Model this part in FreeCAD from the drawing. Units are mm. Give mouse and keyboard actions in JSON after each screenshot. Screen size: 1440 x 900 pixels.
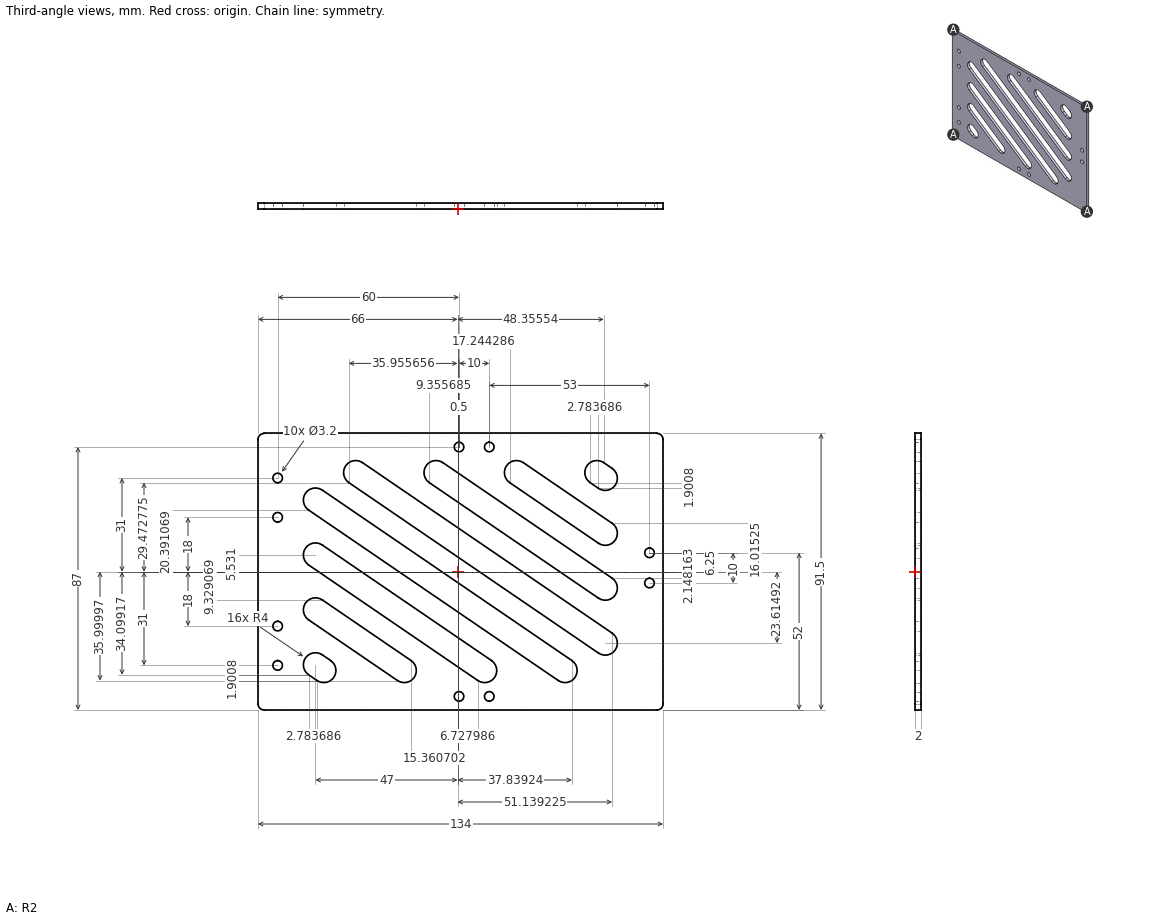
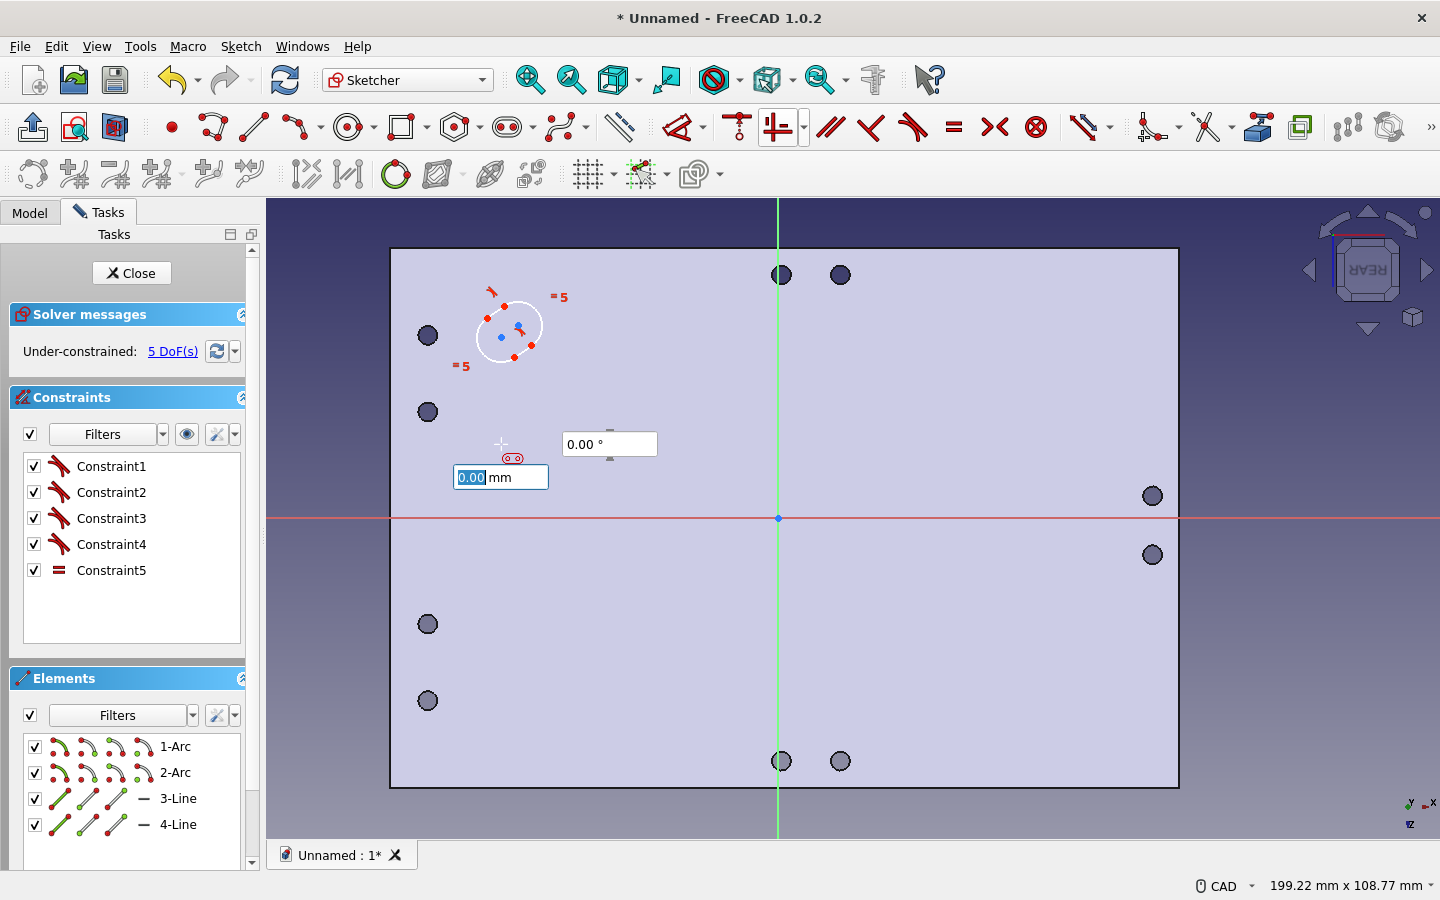
{"action": "left_click", "coordinate": [675, 325]}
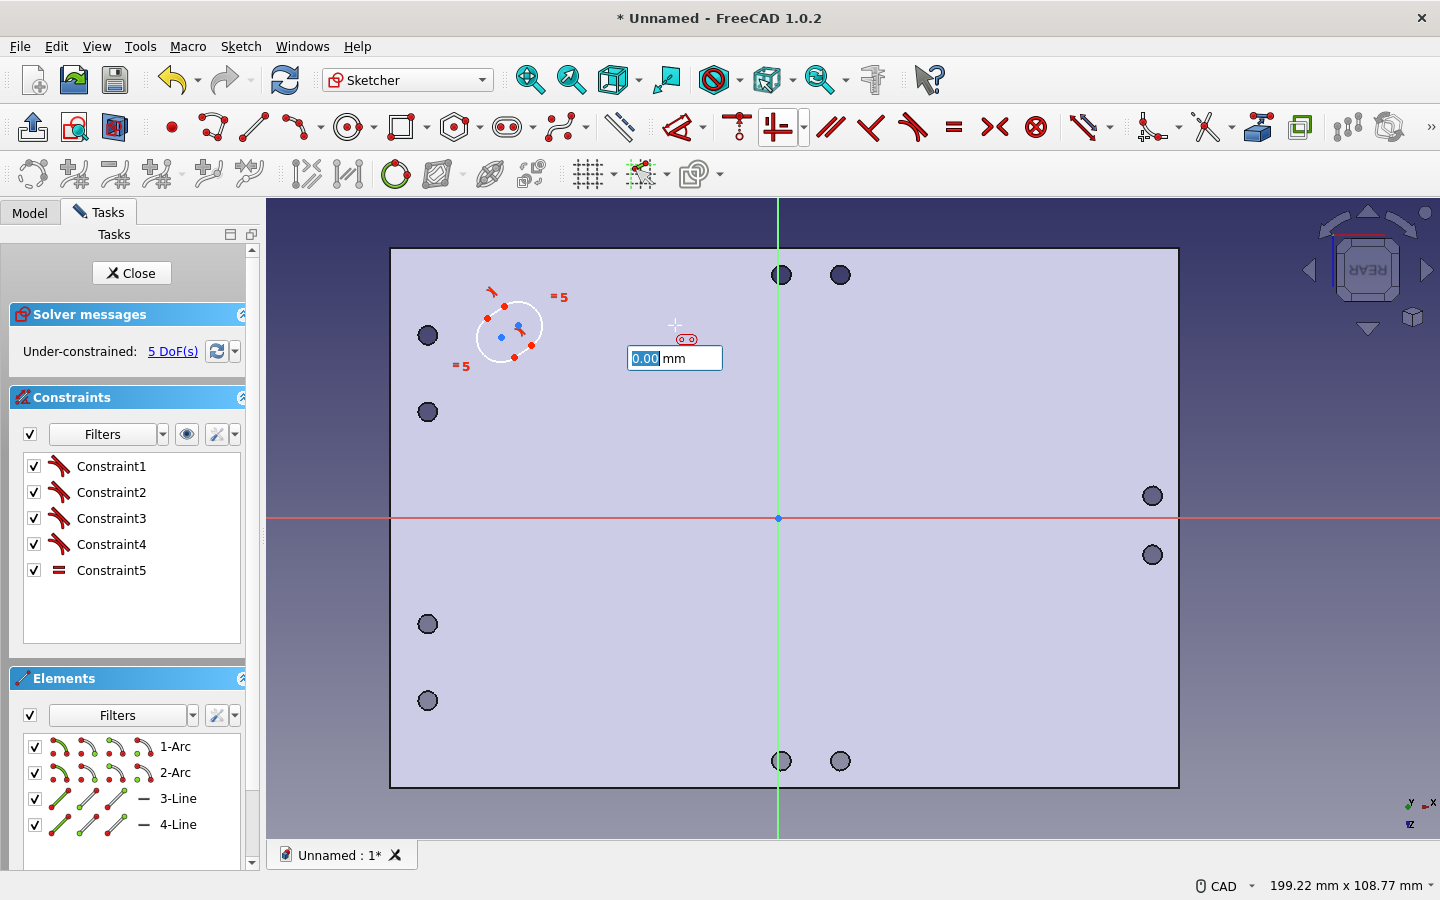
{"action": "left_click", "coordinate": [575, 365]}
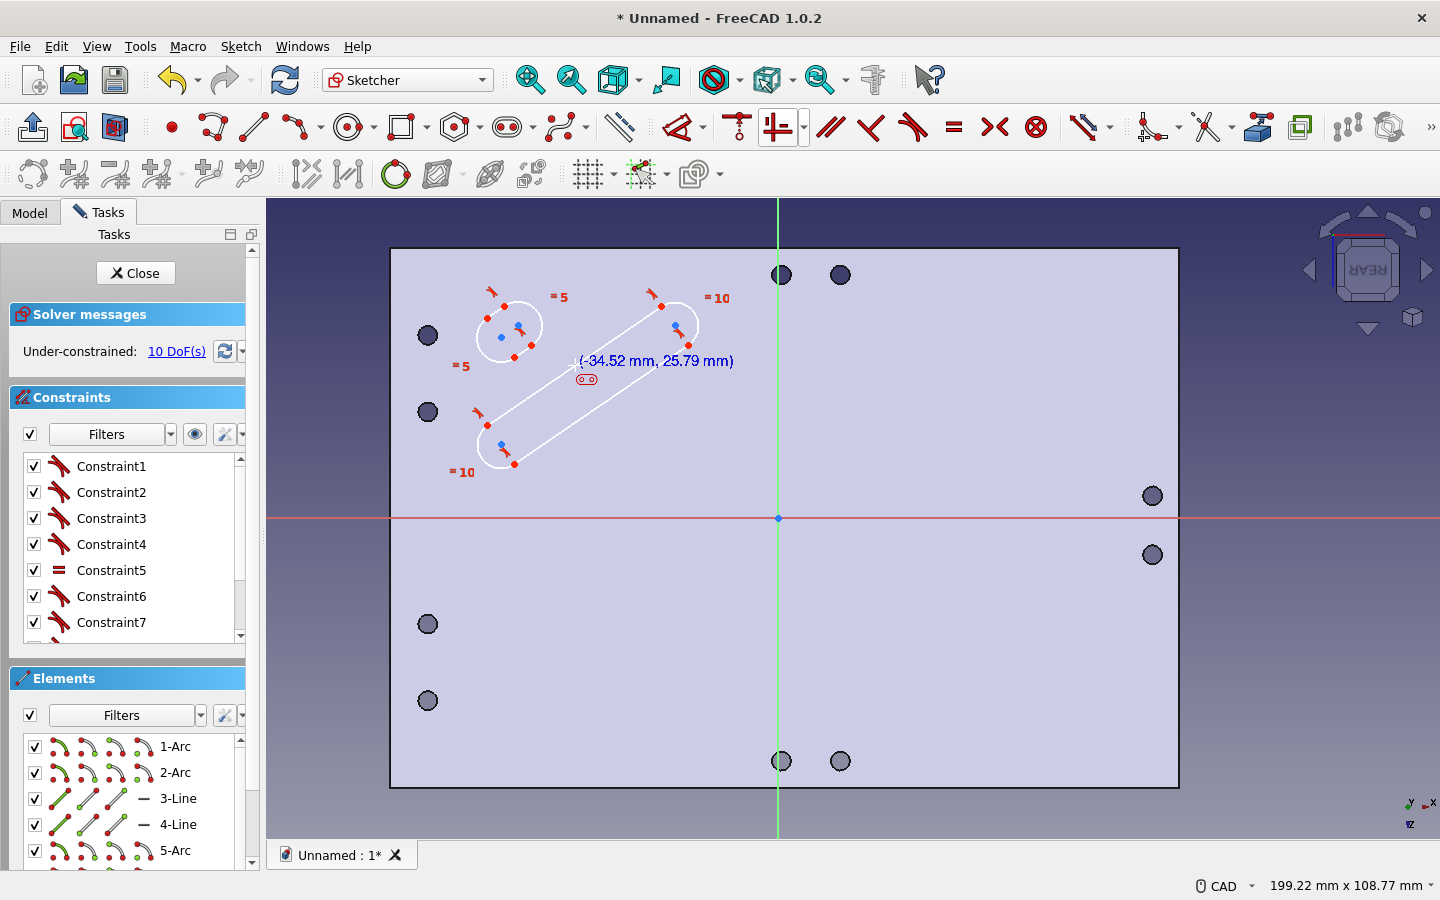
{"action": "left_click", "coordinate": [501, 551]}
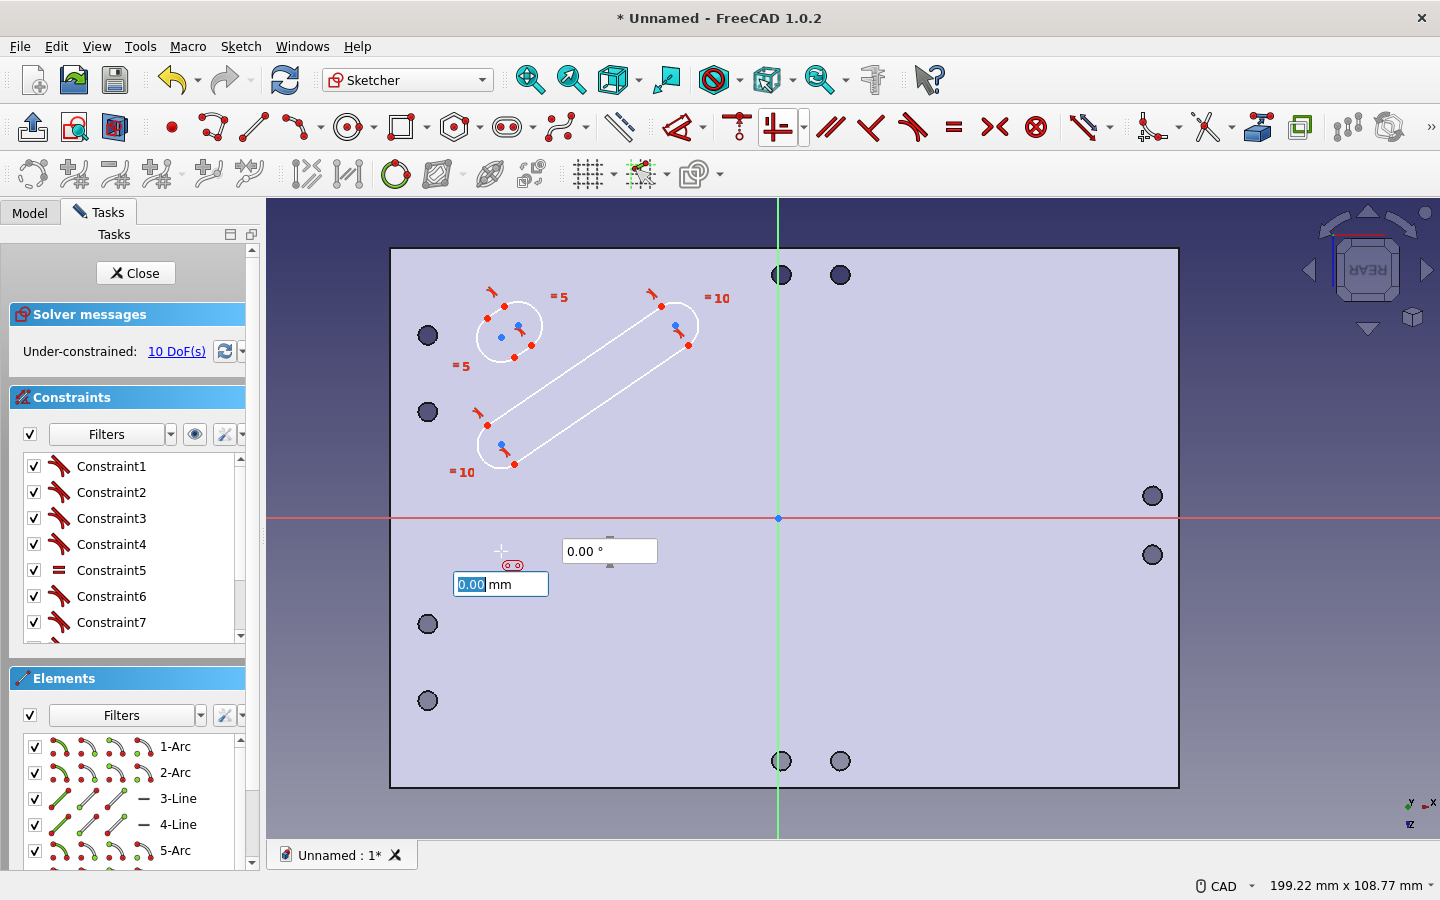
{"action": "left_click", "coordinate": [831, 325]}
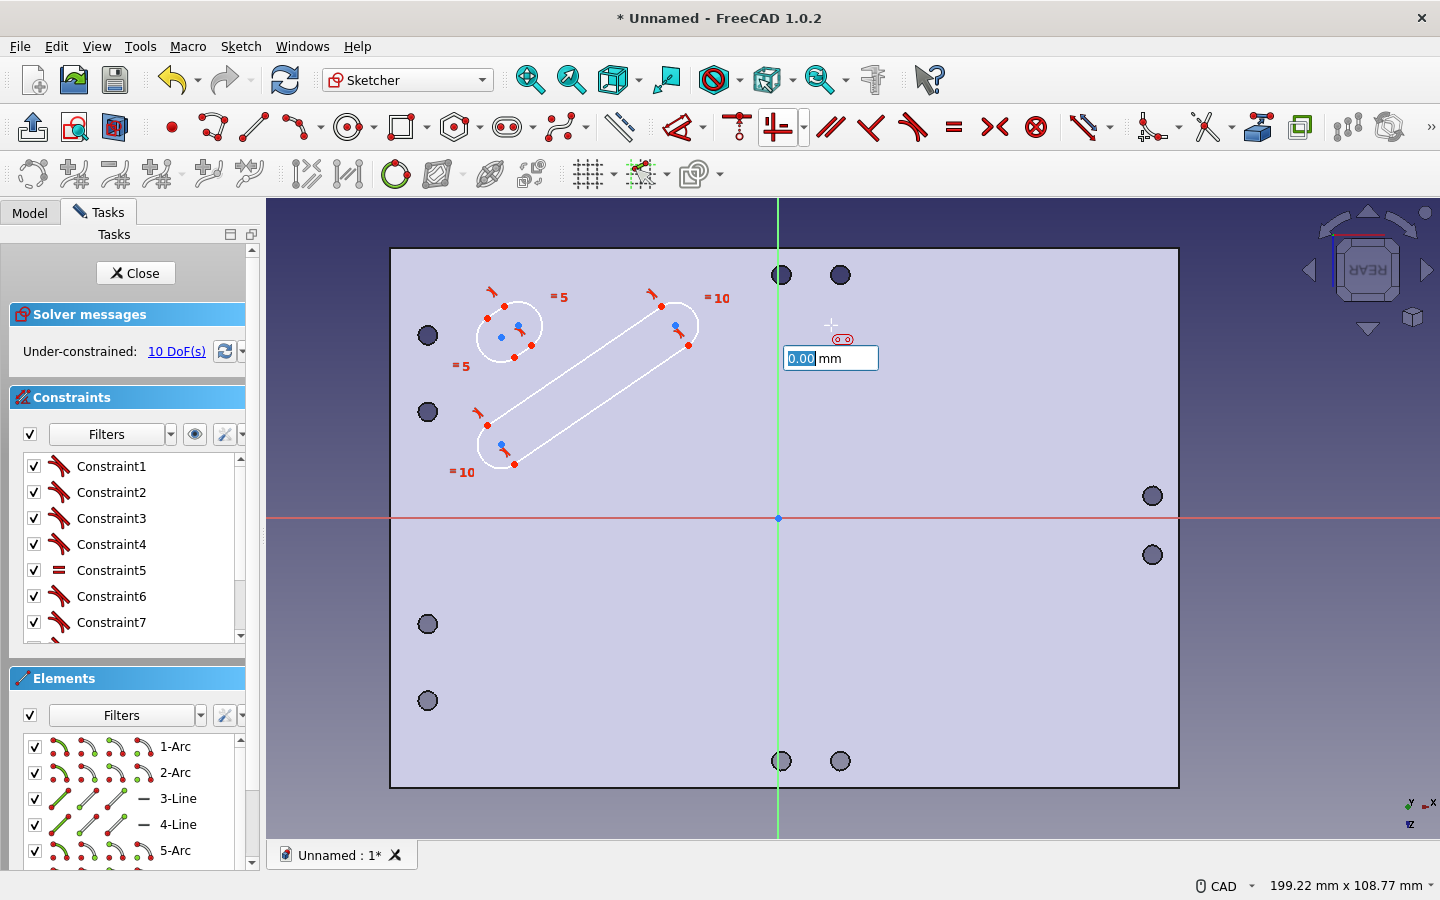
{"action": "left_click", "coordinate": [653, 418]}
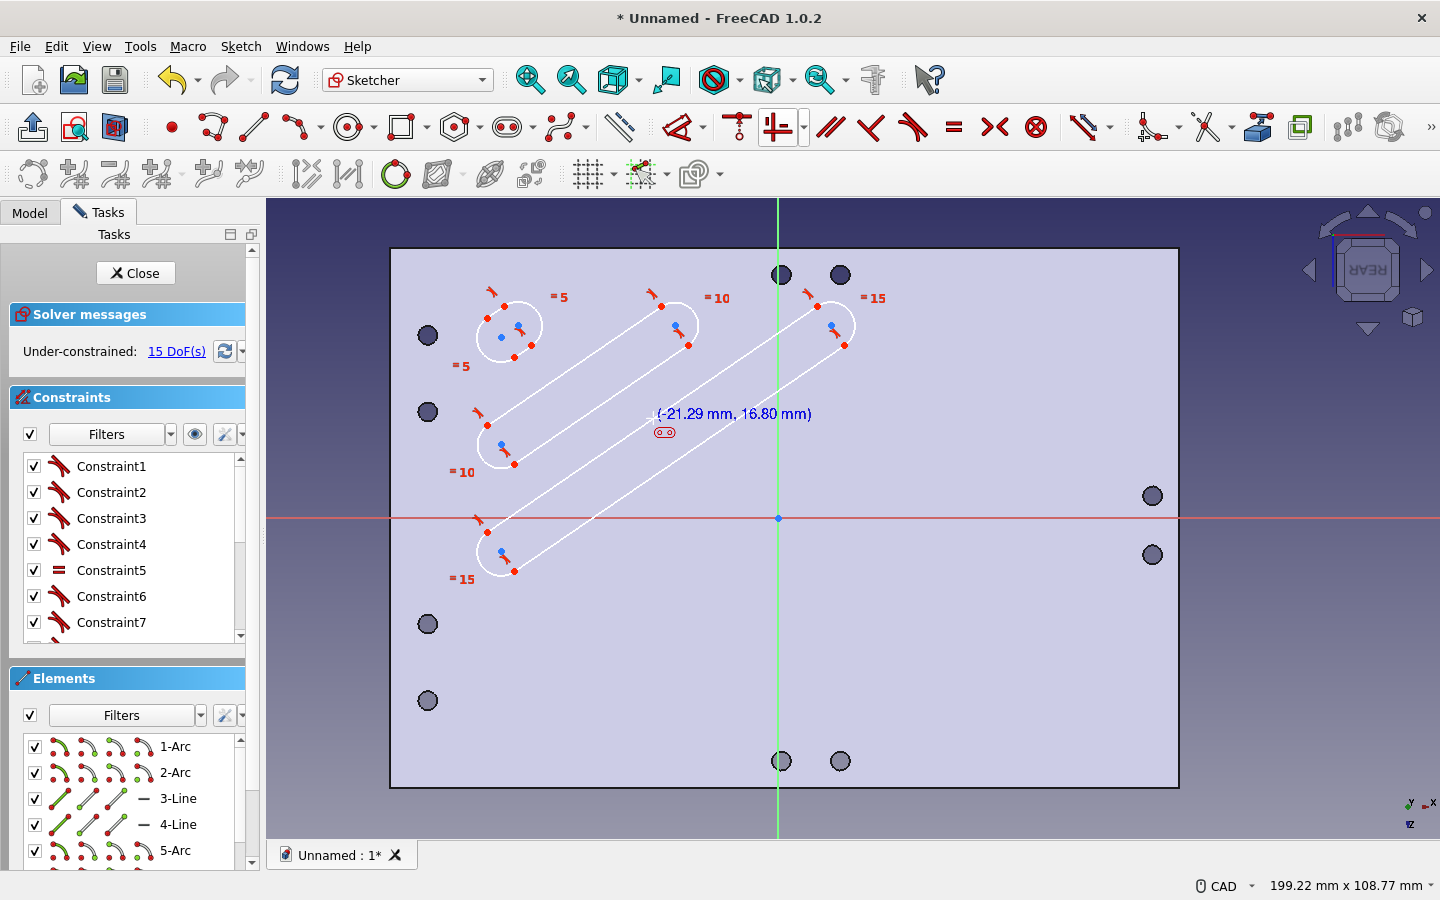
{"action": "left_click", "coordinate": [501, 658]}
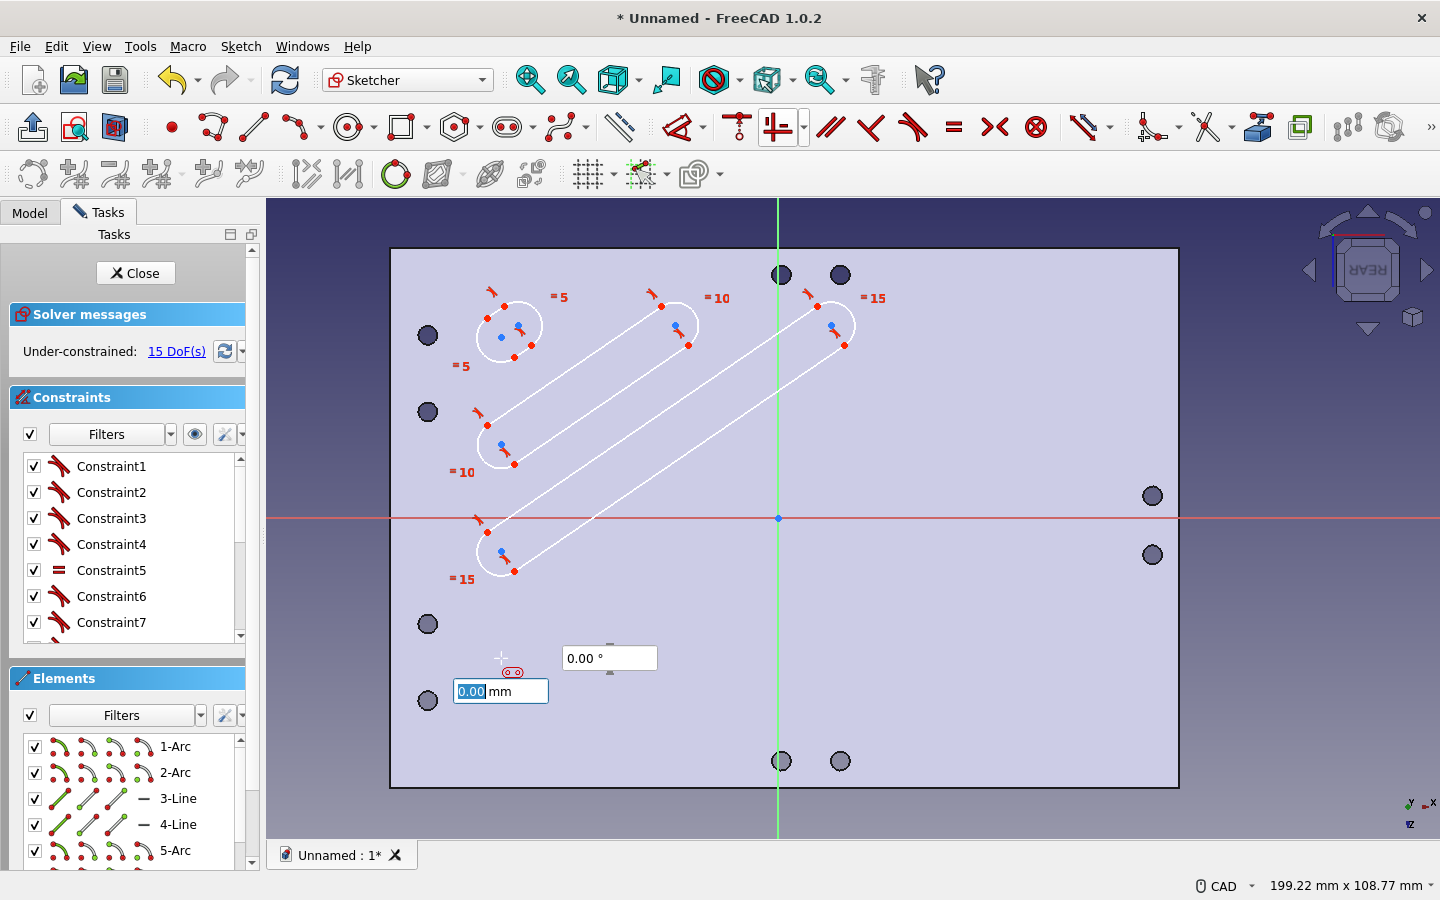
{"action": "left_click", "coordinate": [988, 325]}